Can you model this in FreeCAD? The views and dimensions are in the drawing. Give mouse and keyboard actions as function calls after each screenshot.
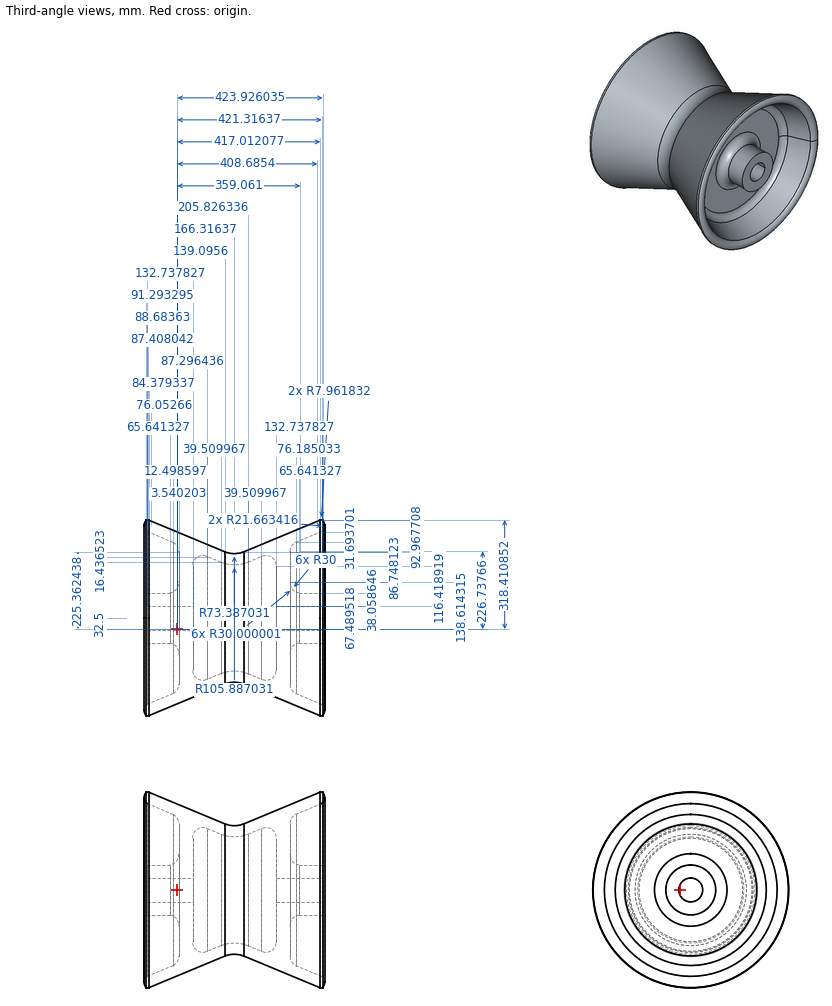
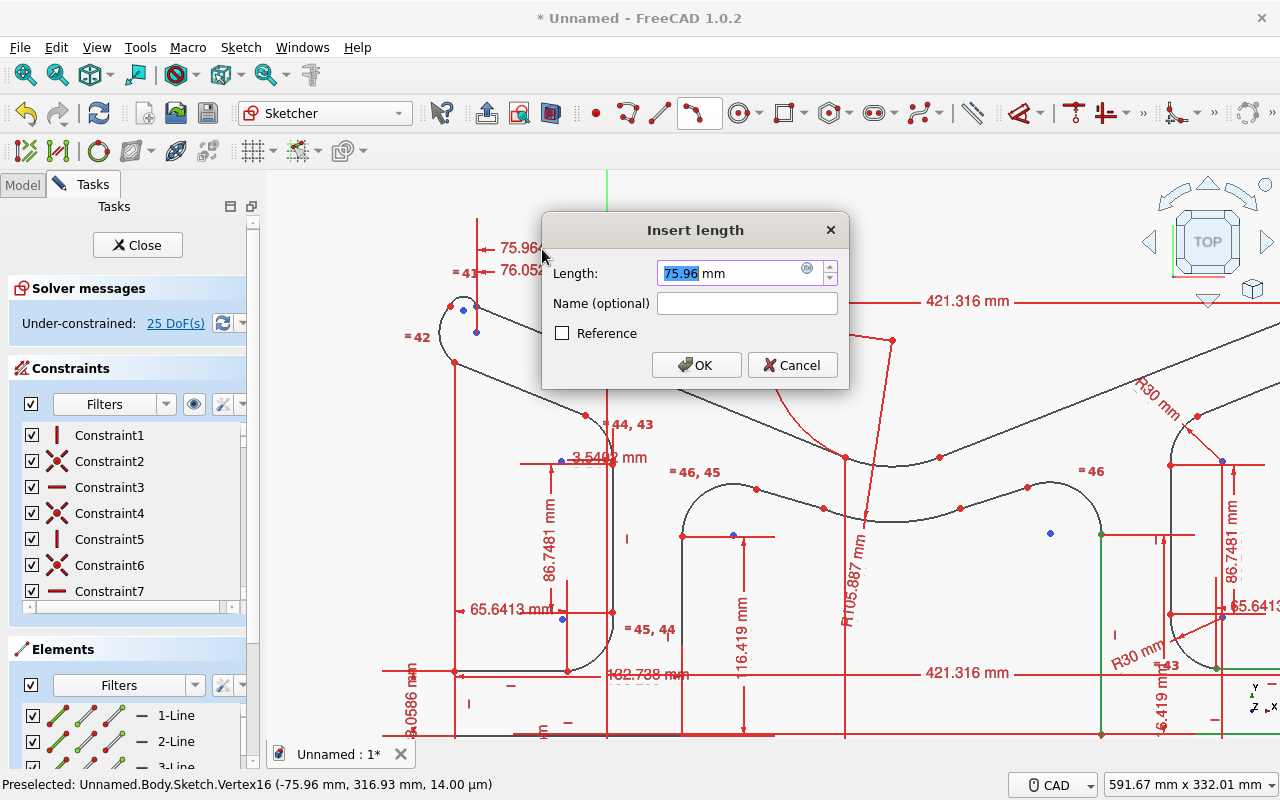
text(84.379337)
key(Return)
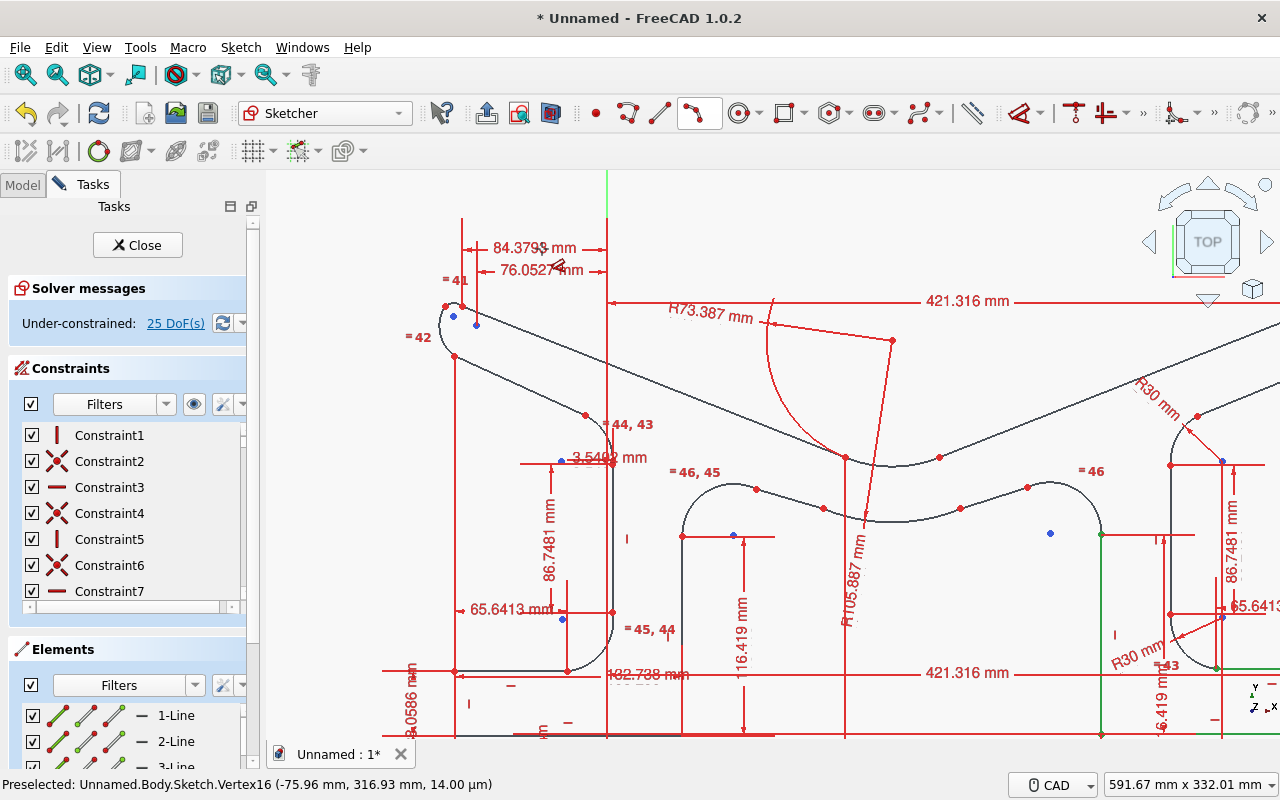
scroll(586, 416, up, 4)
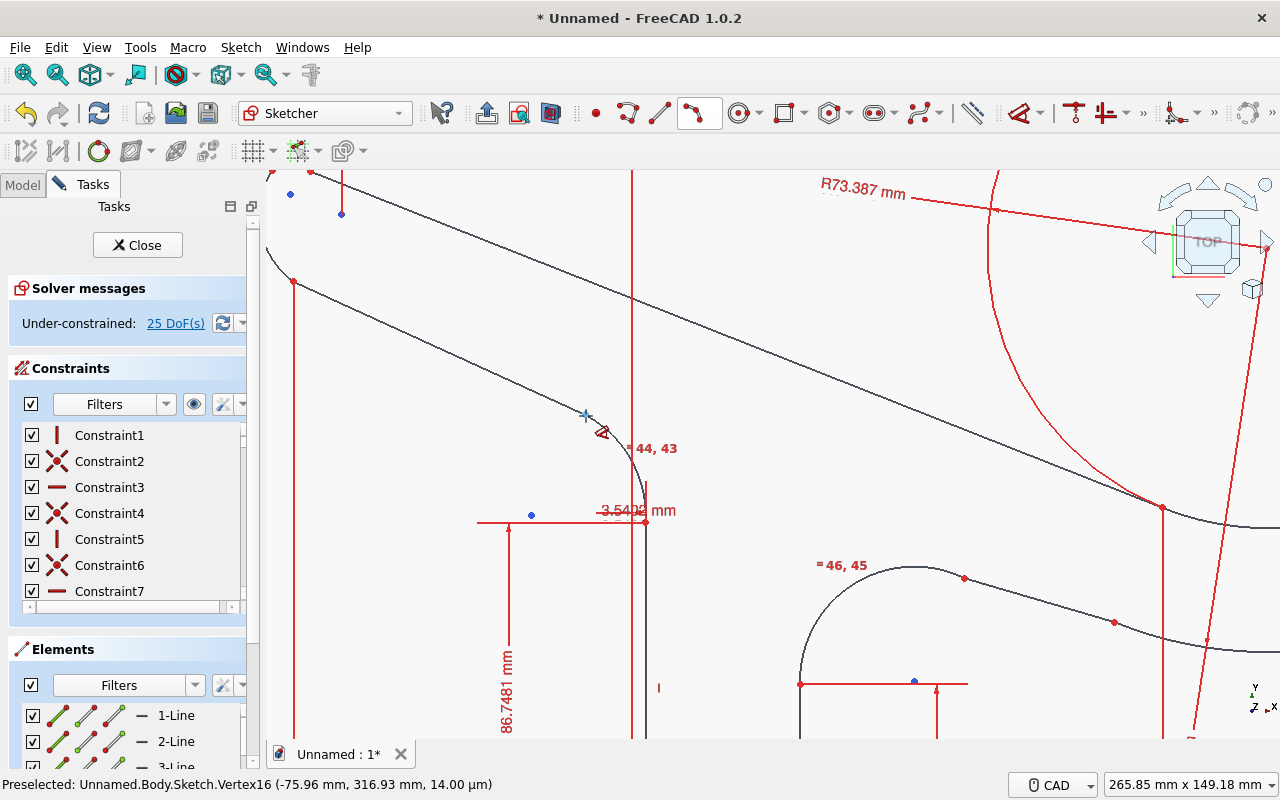
click(585, 415)
click(609, 381)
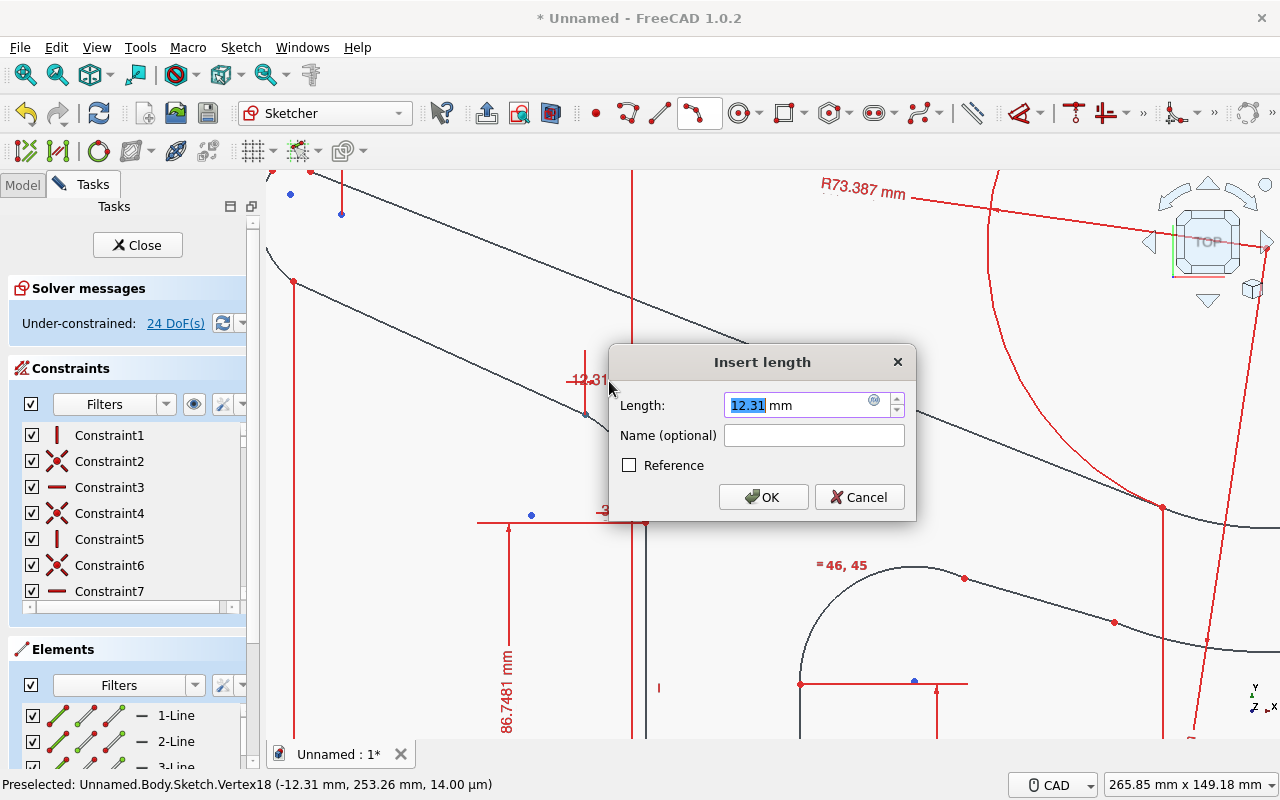
text(12.498597)
key(Return)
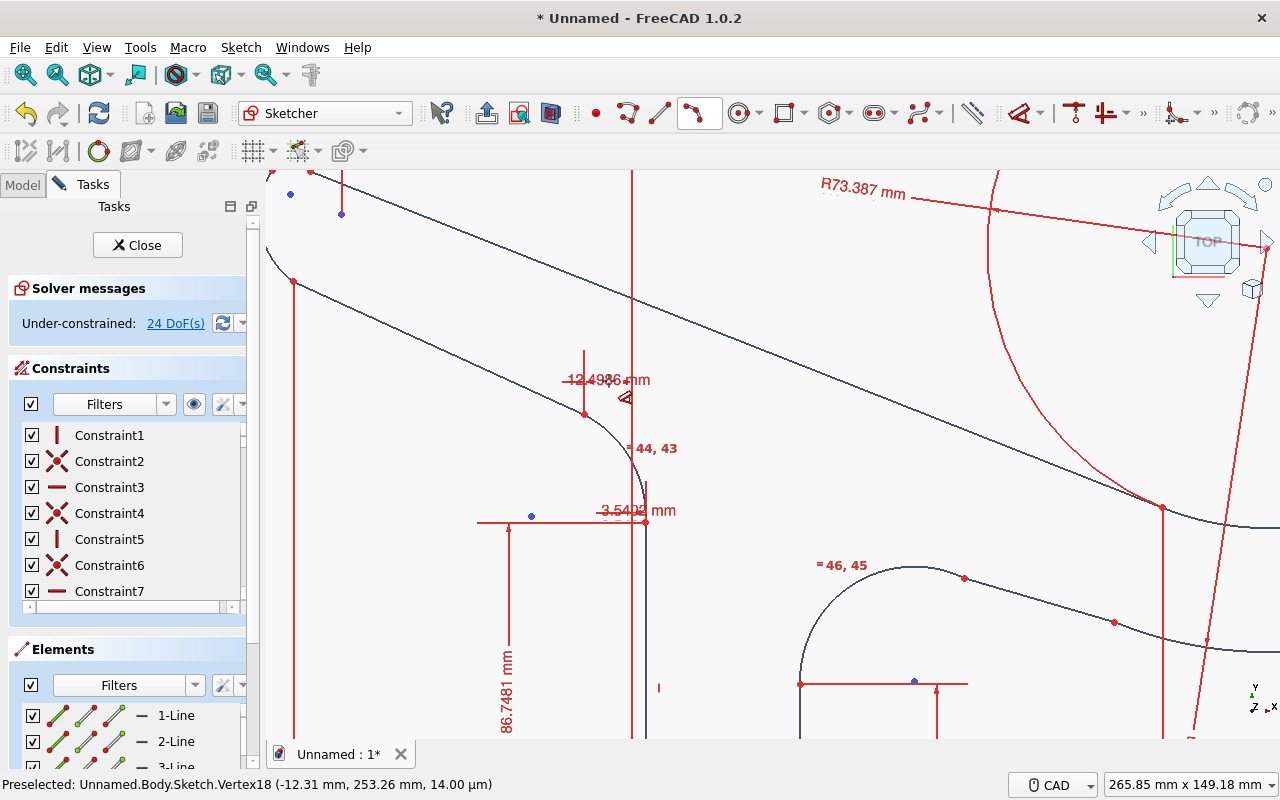
scroll(521, 350, down, 7)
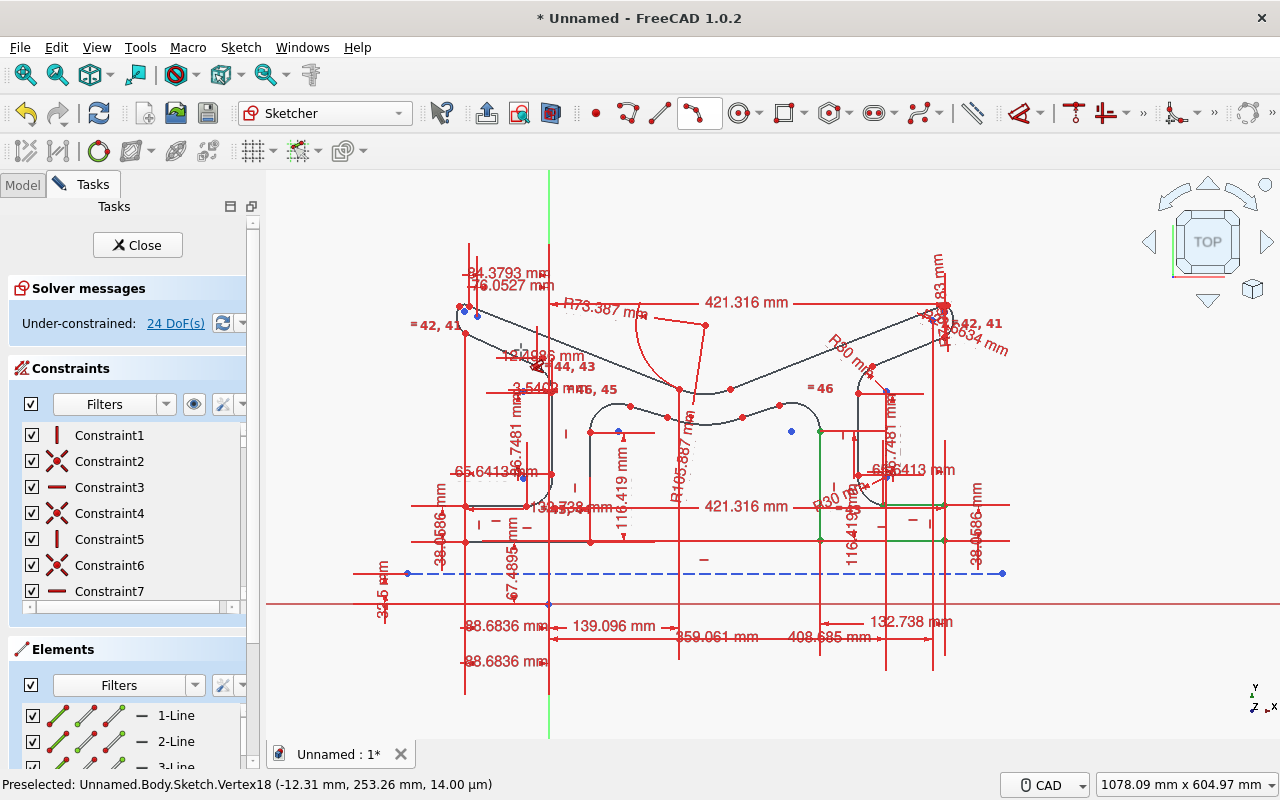
click(465, 542)
click(431, 559)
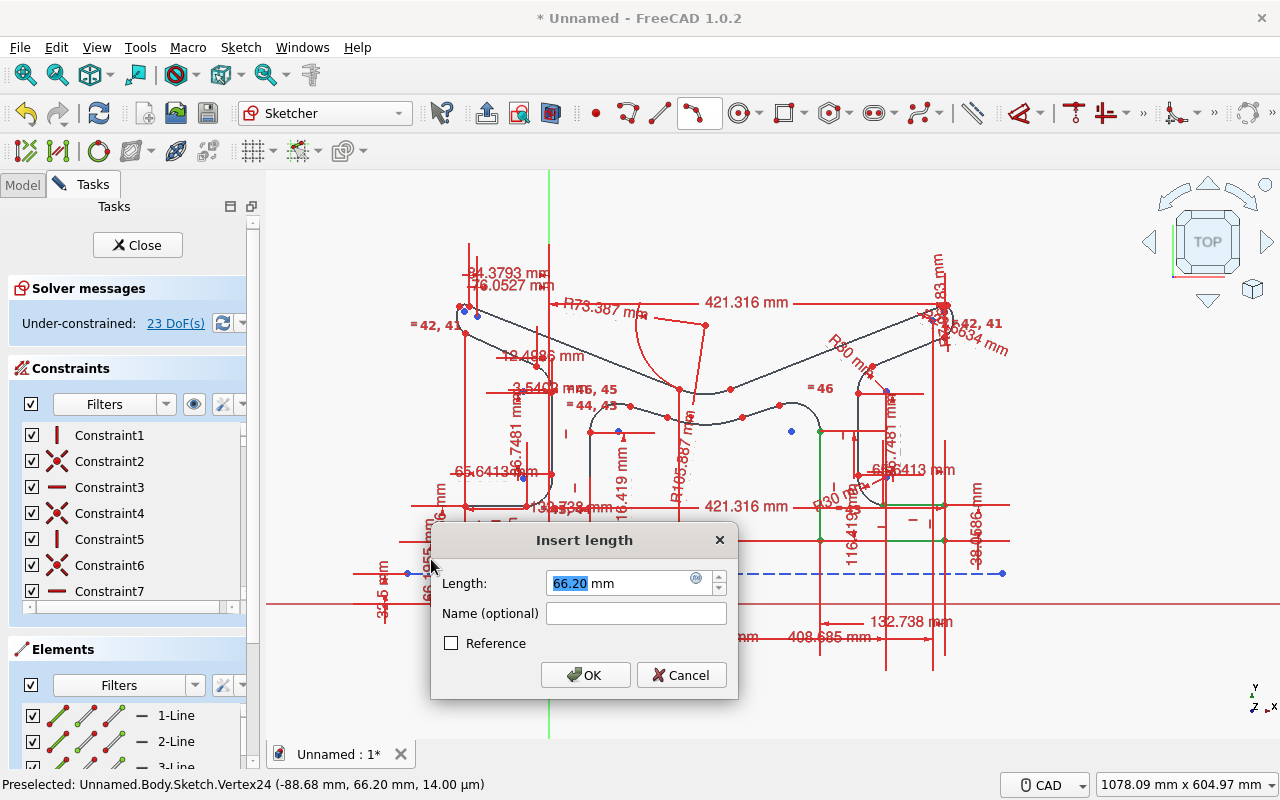
text(67.489518)
key(Return)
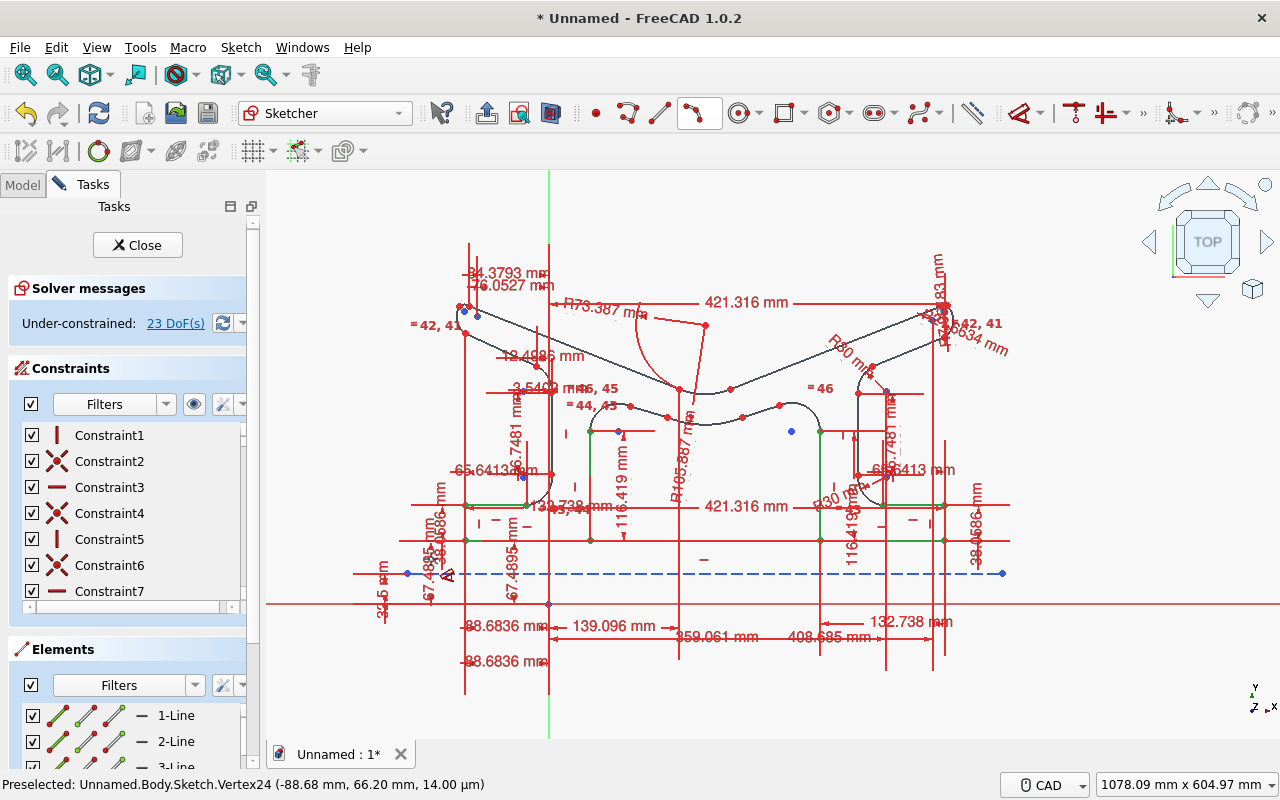
click(631, 407)
click(590, 662)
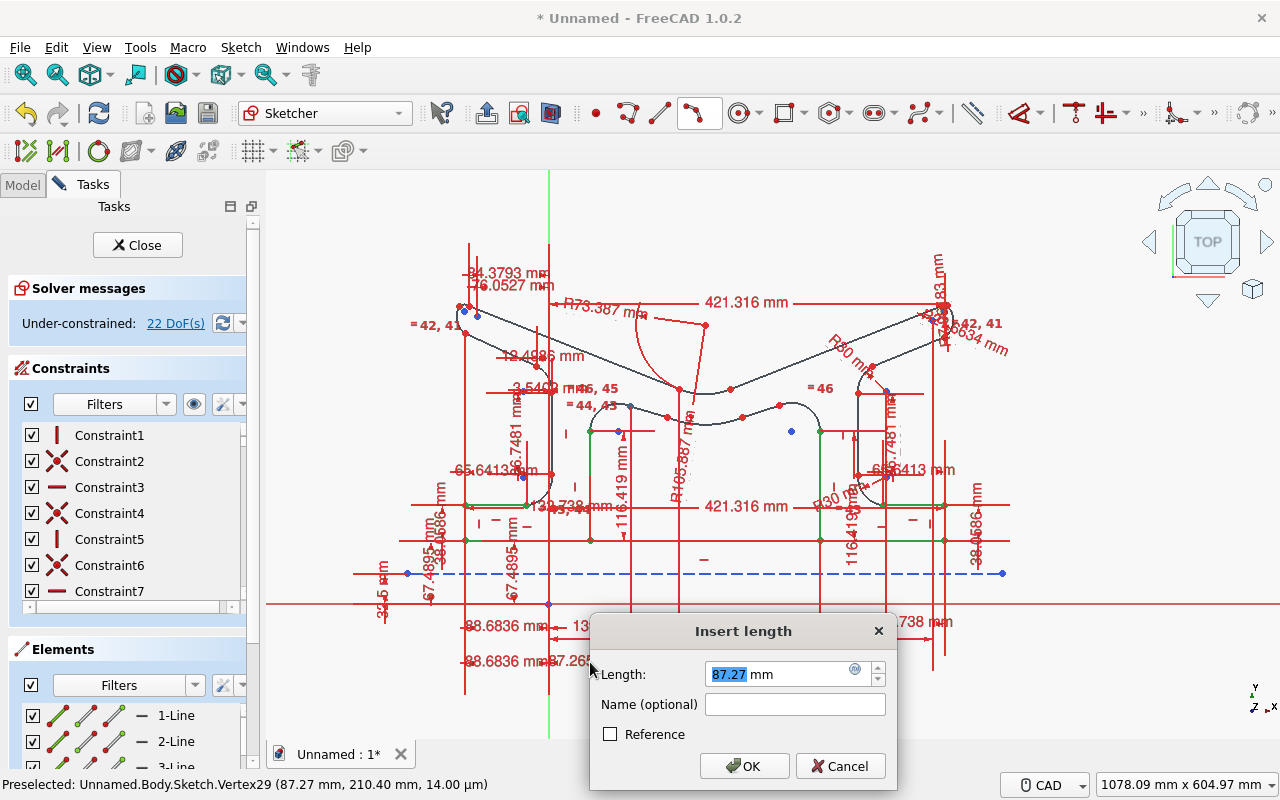
text(87.296436)
key(Return)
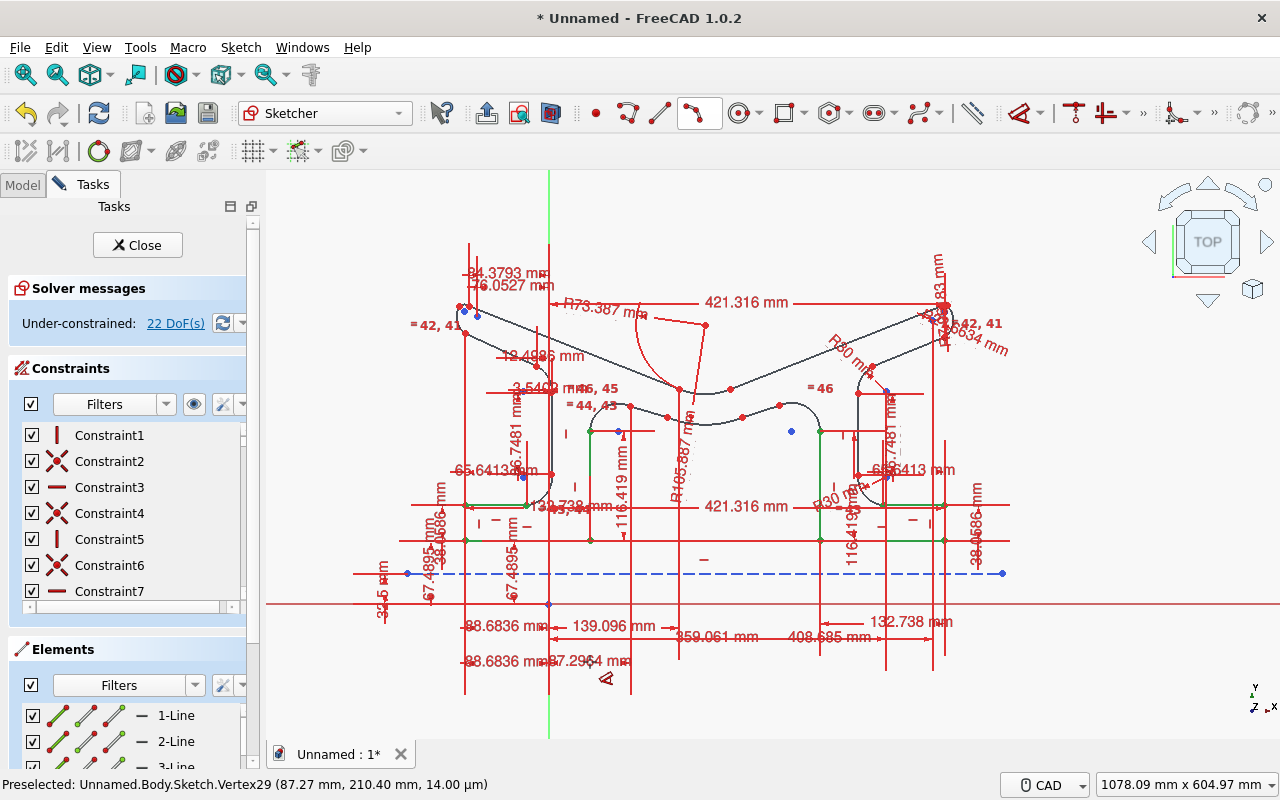
scroll(460, 306, up, 3)